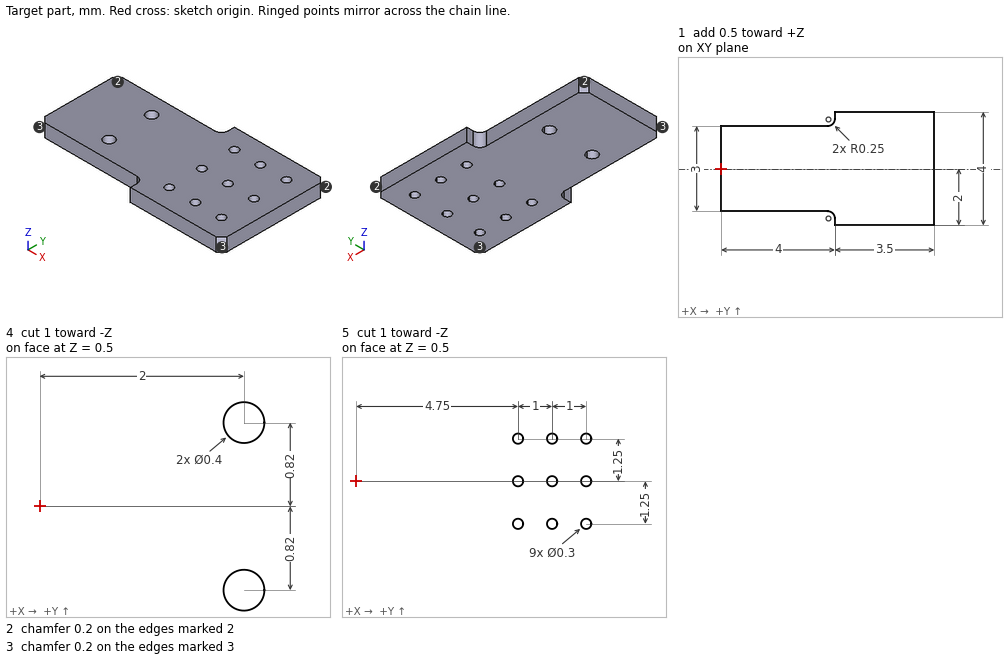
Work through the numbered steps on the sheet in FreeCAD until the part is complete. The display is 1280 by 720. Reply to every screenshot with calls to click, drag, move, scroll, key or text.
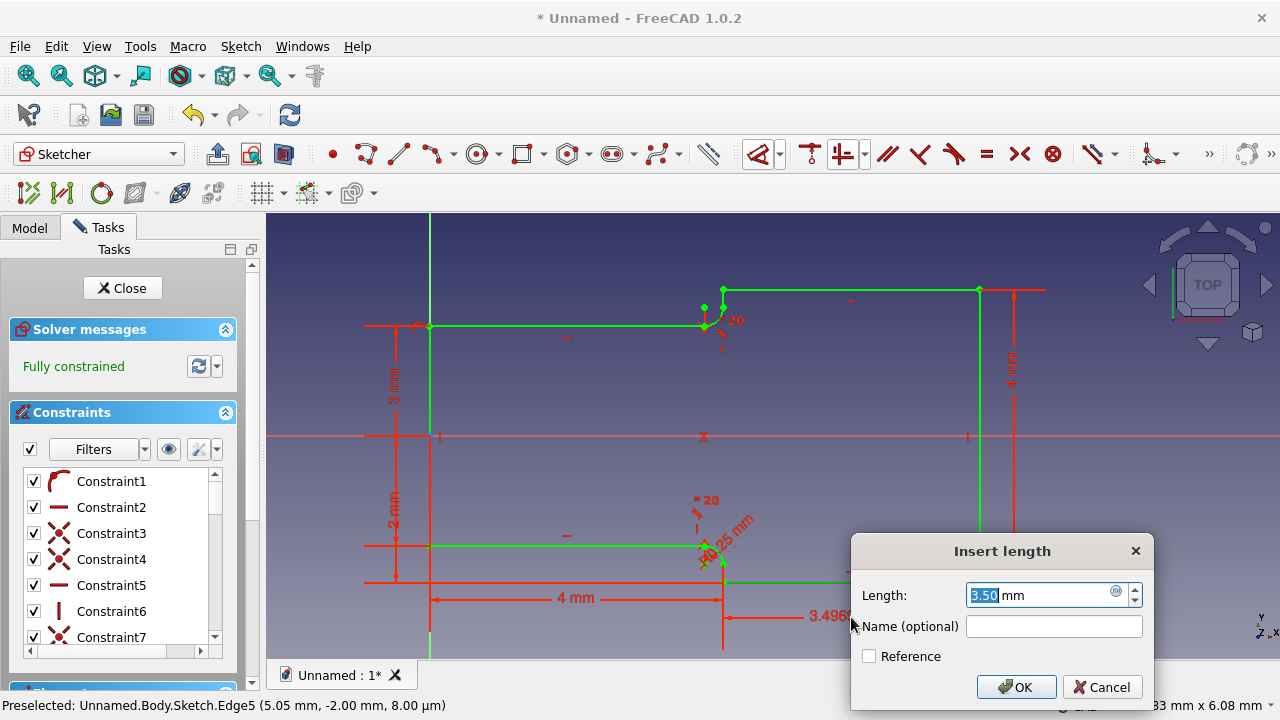
text(3.5)
key(Return)
key(Escape)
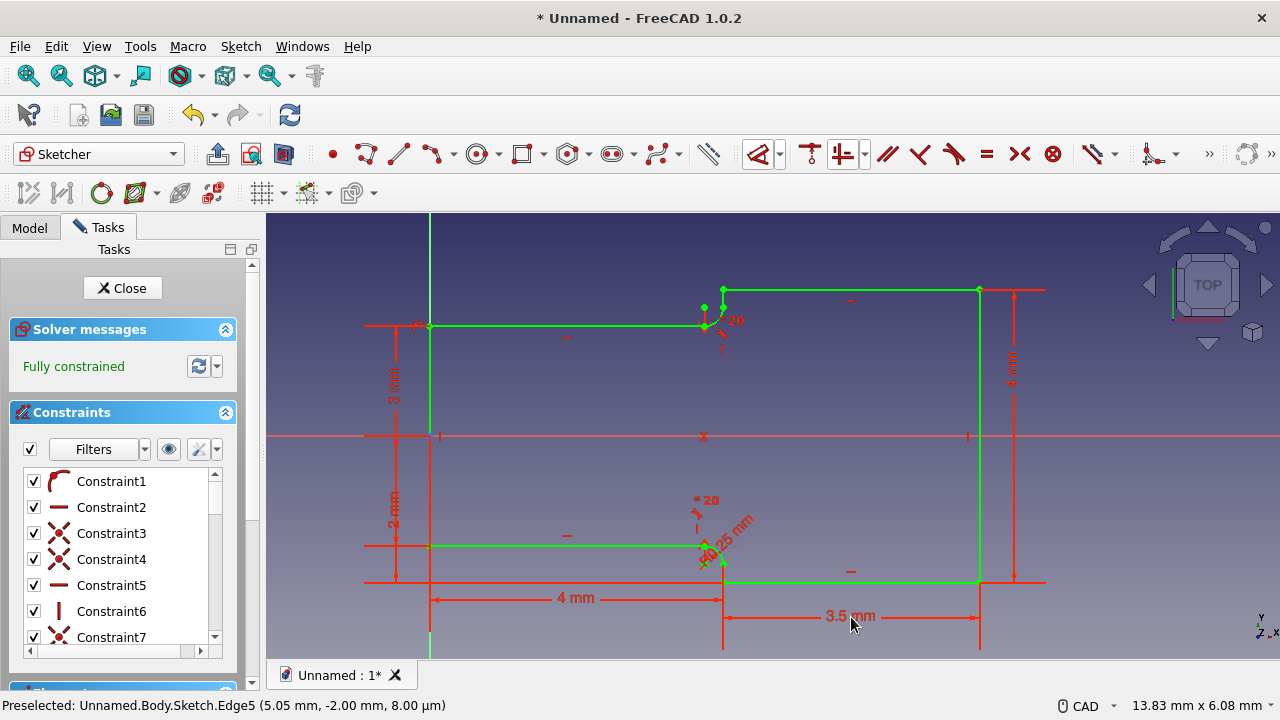
click(123, 288)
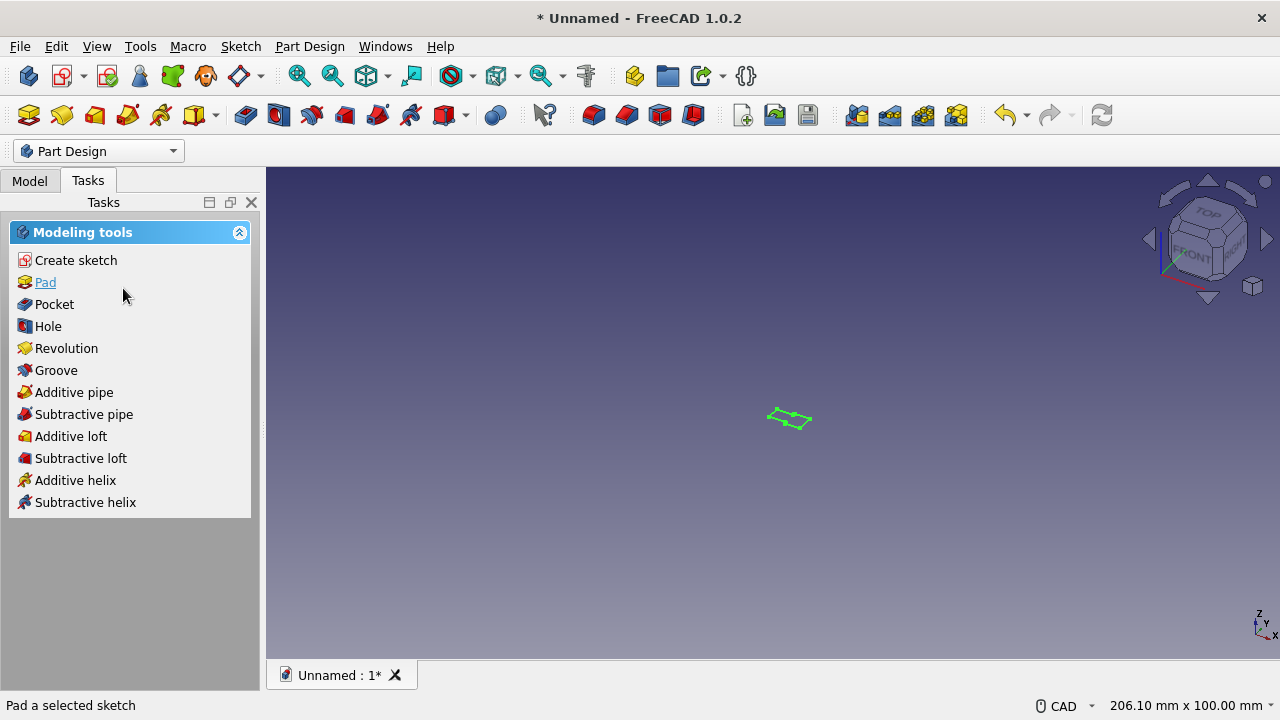
click(29, 116)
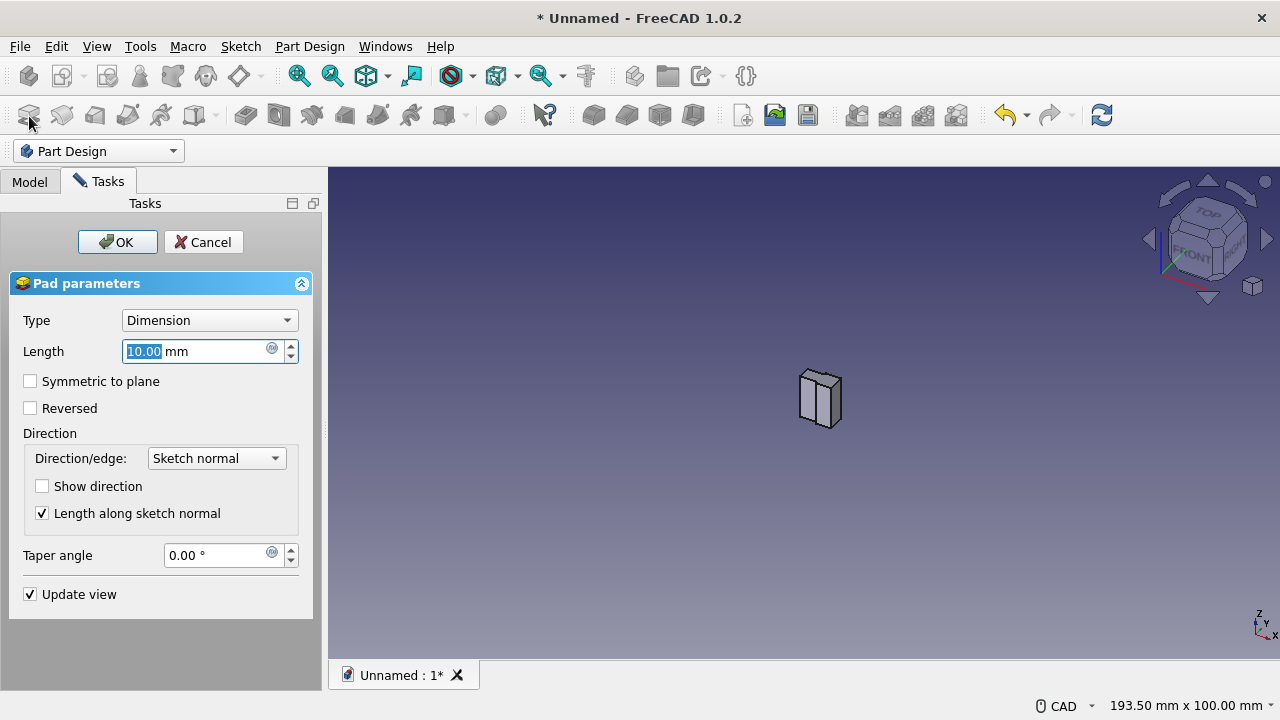
text(0.5)
key(Tab)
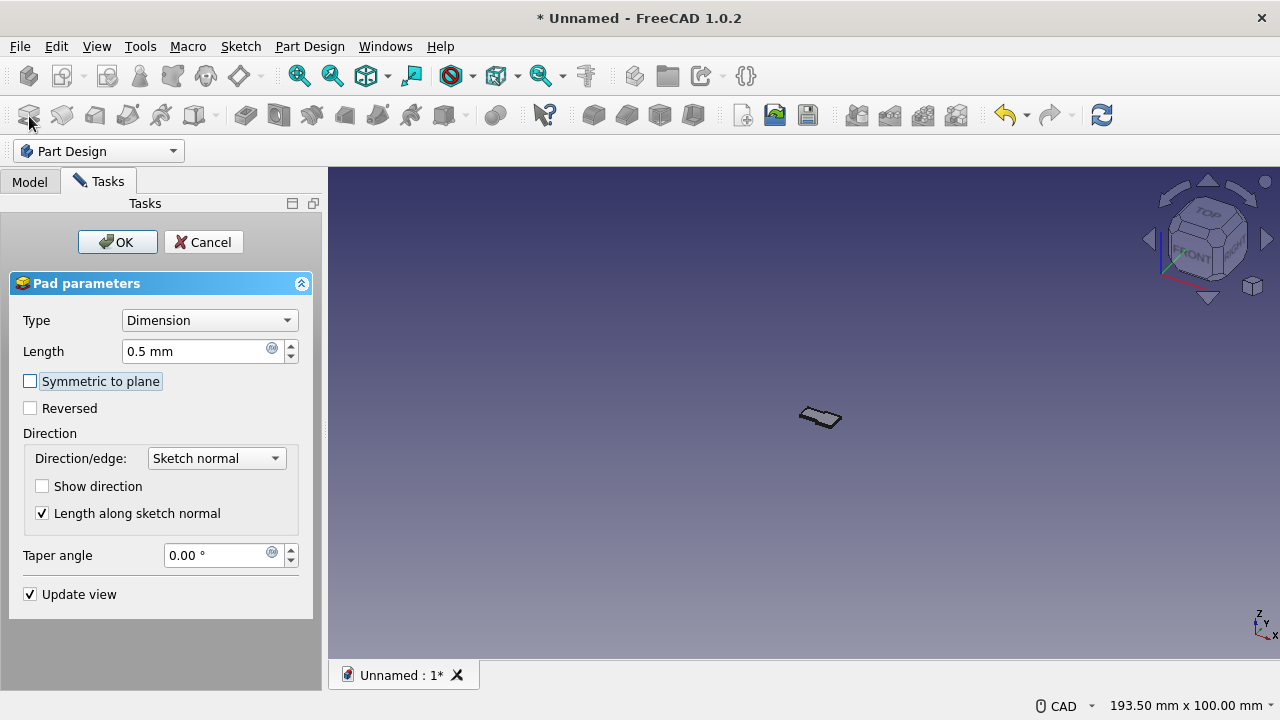
click(118, 242)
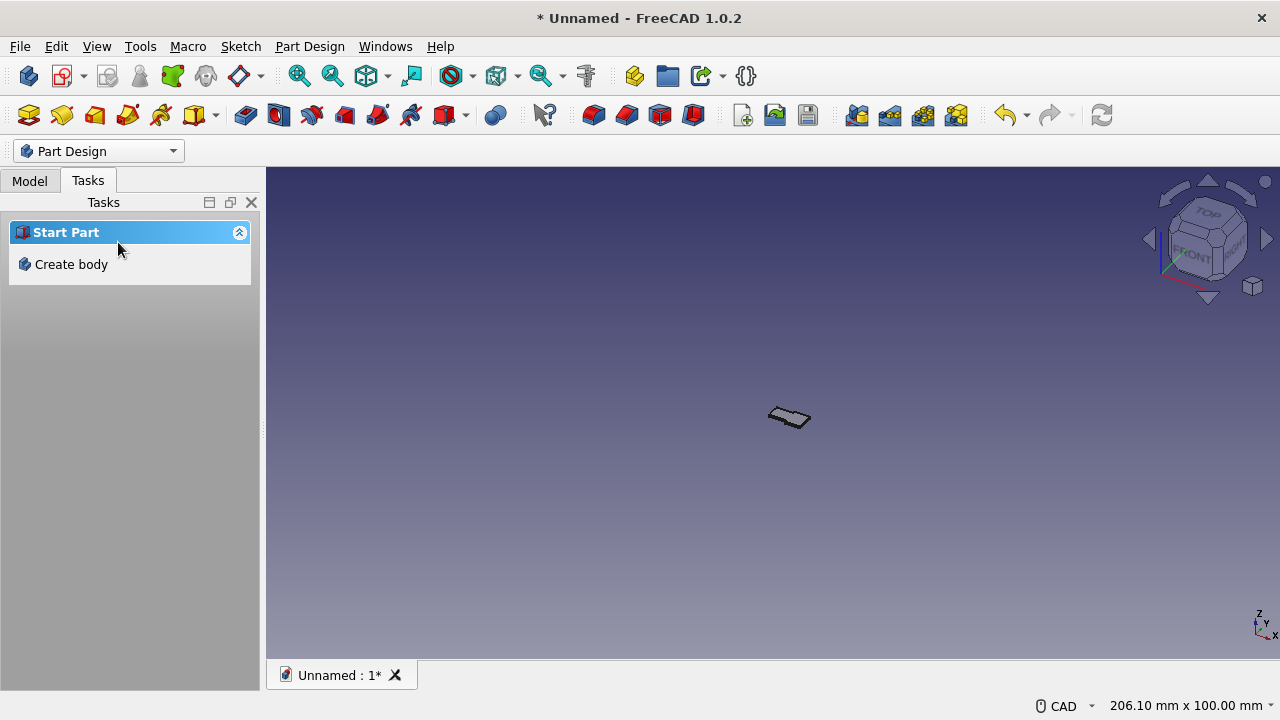
key(v)
key(f)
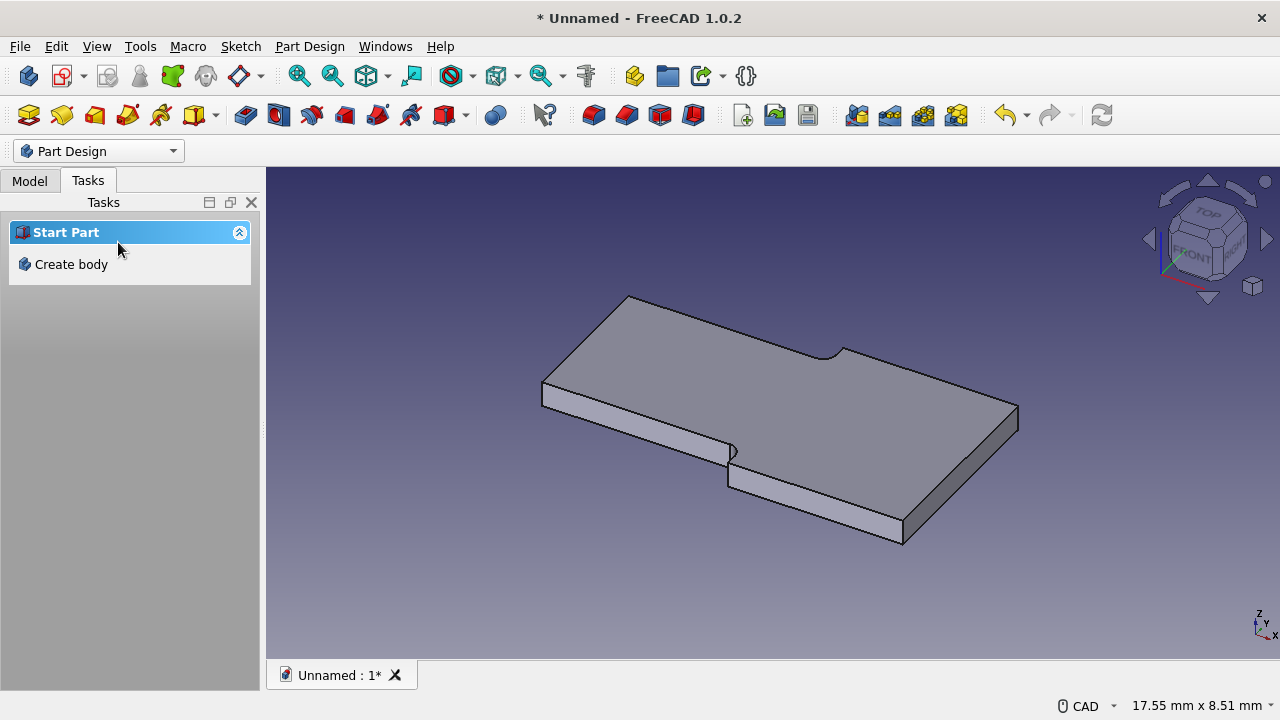
key(0)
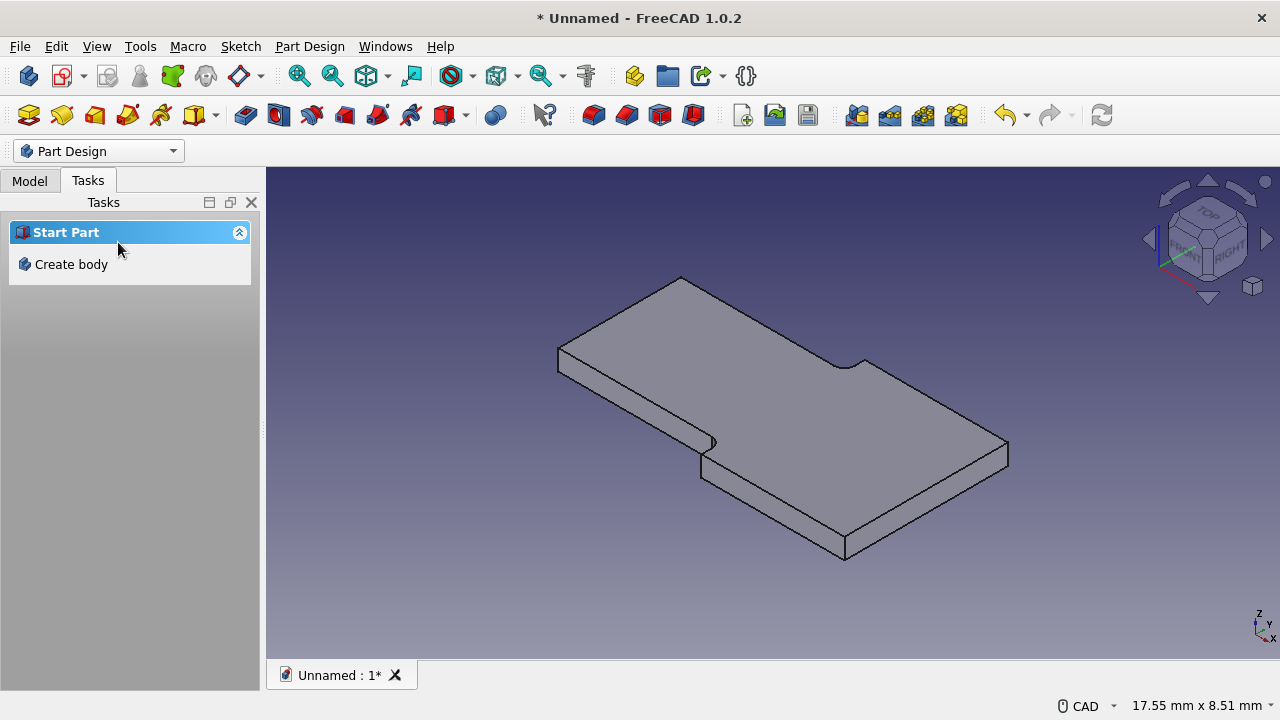
key(2)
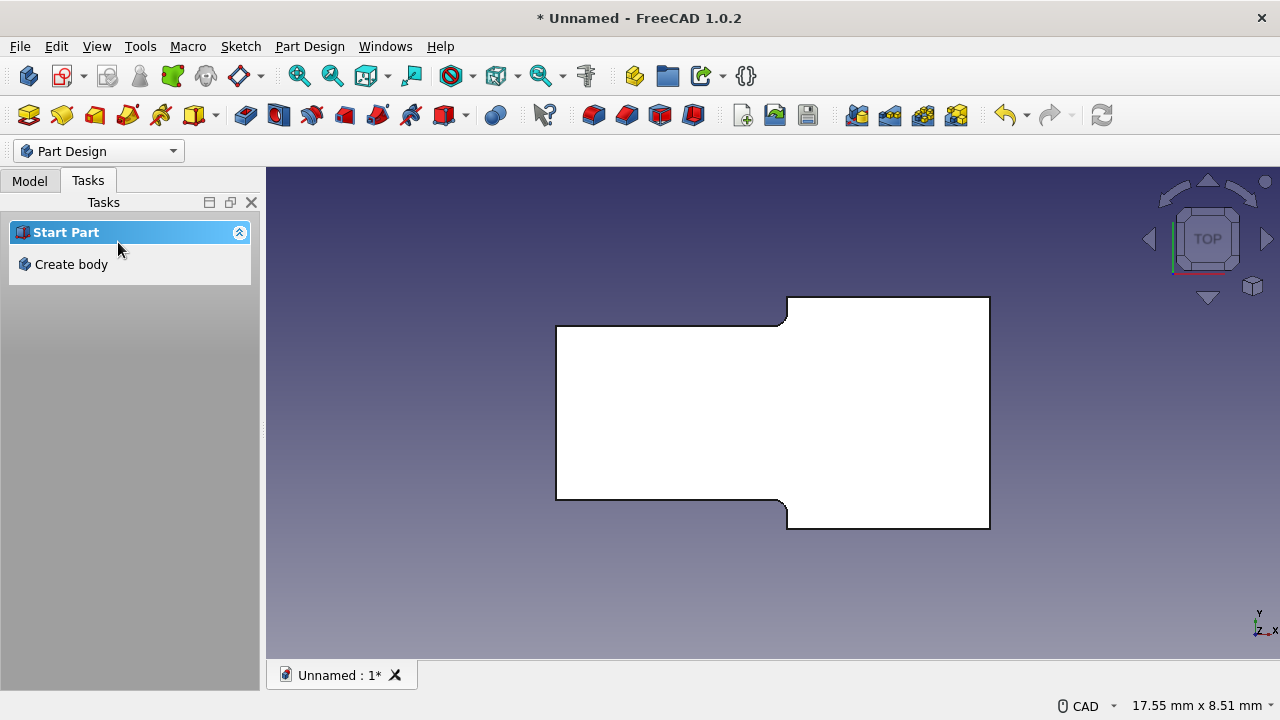
key(1)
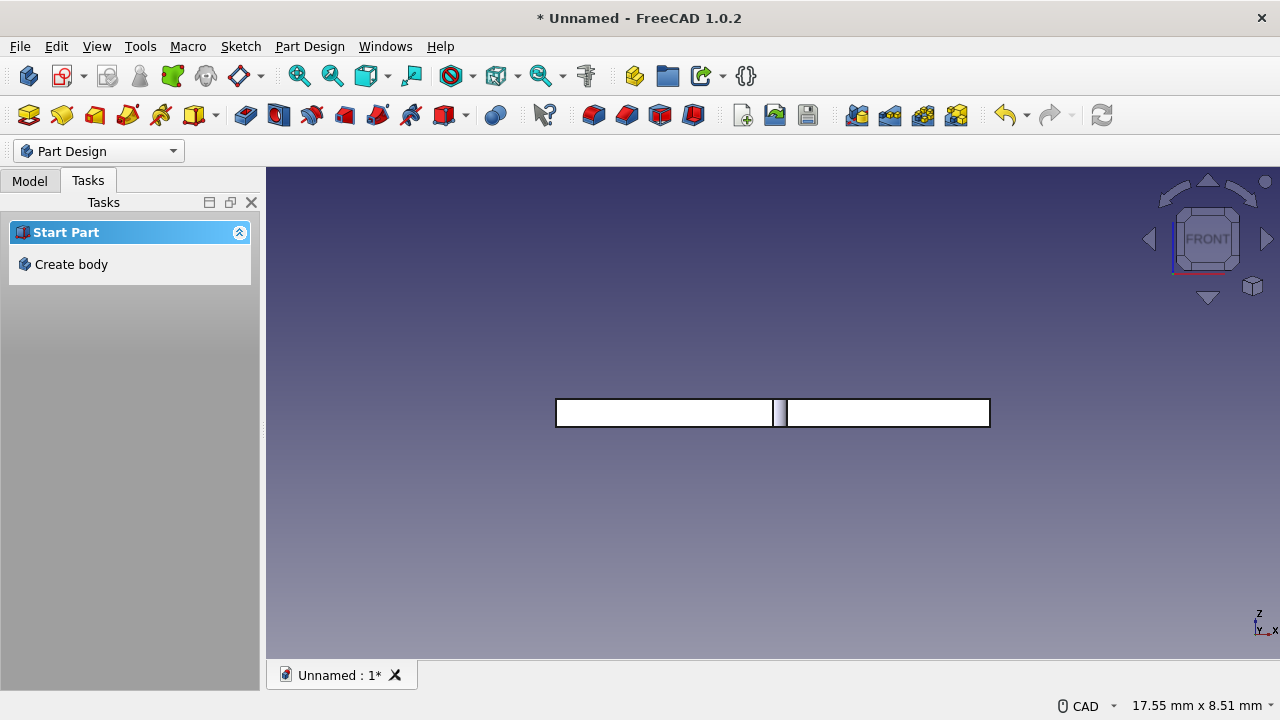
click(300, 76)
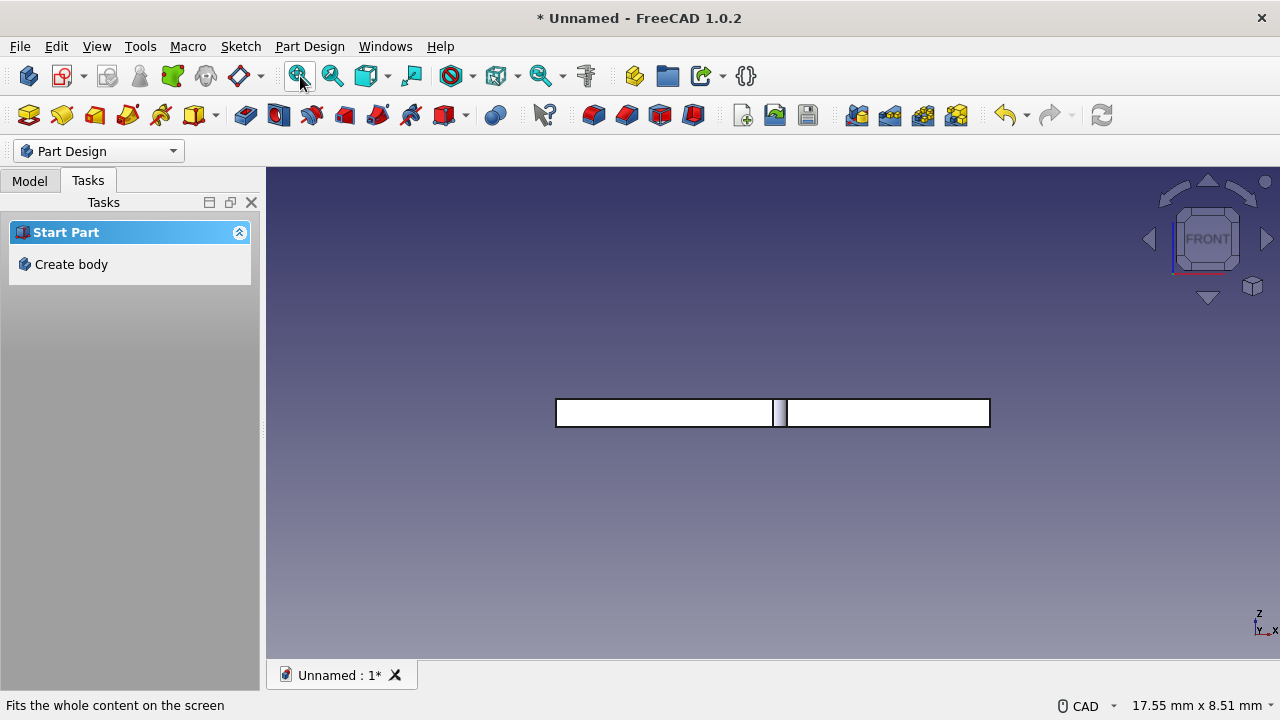
key(3)